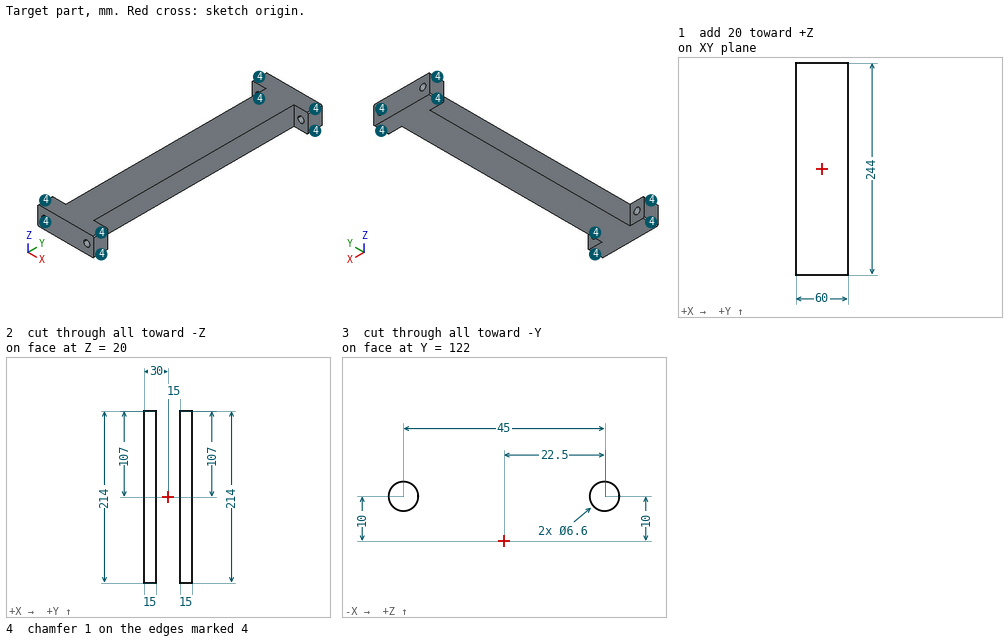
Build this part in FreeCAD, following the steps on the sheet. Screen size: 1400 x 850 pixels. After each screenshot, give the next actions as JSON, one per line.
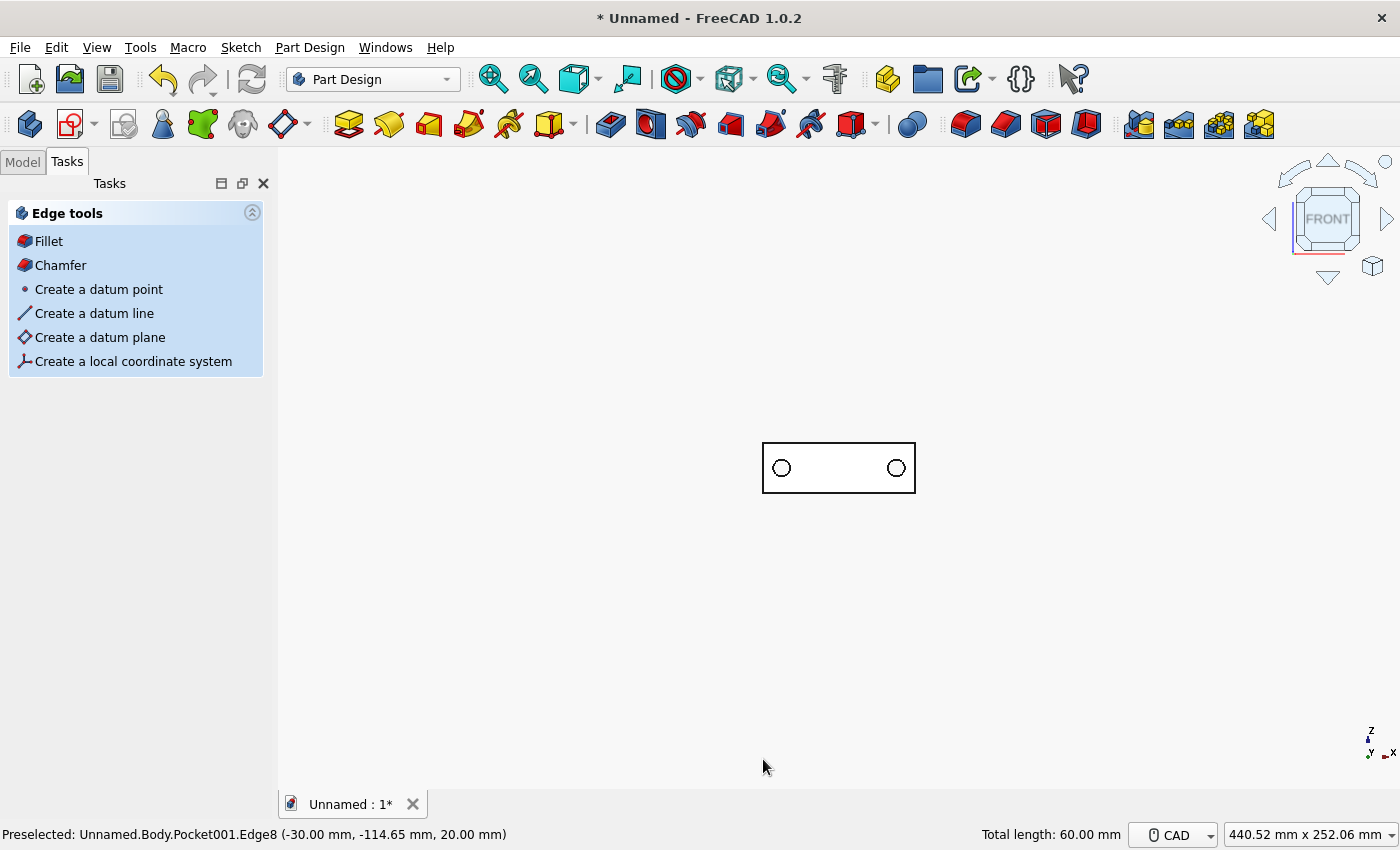
{"action": "left_click", "coordinate": [494, 80]}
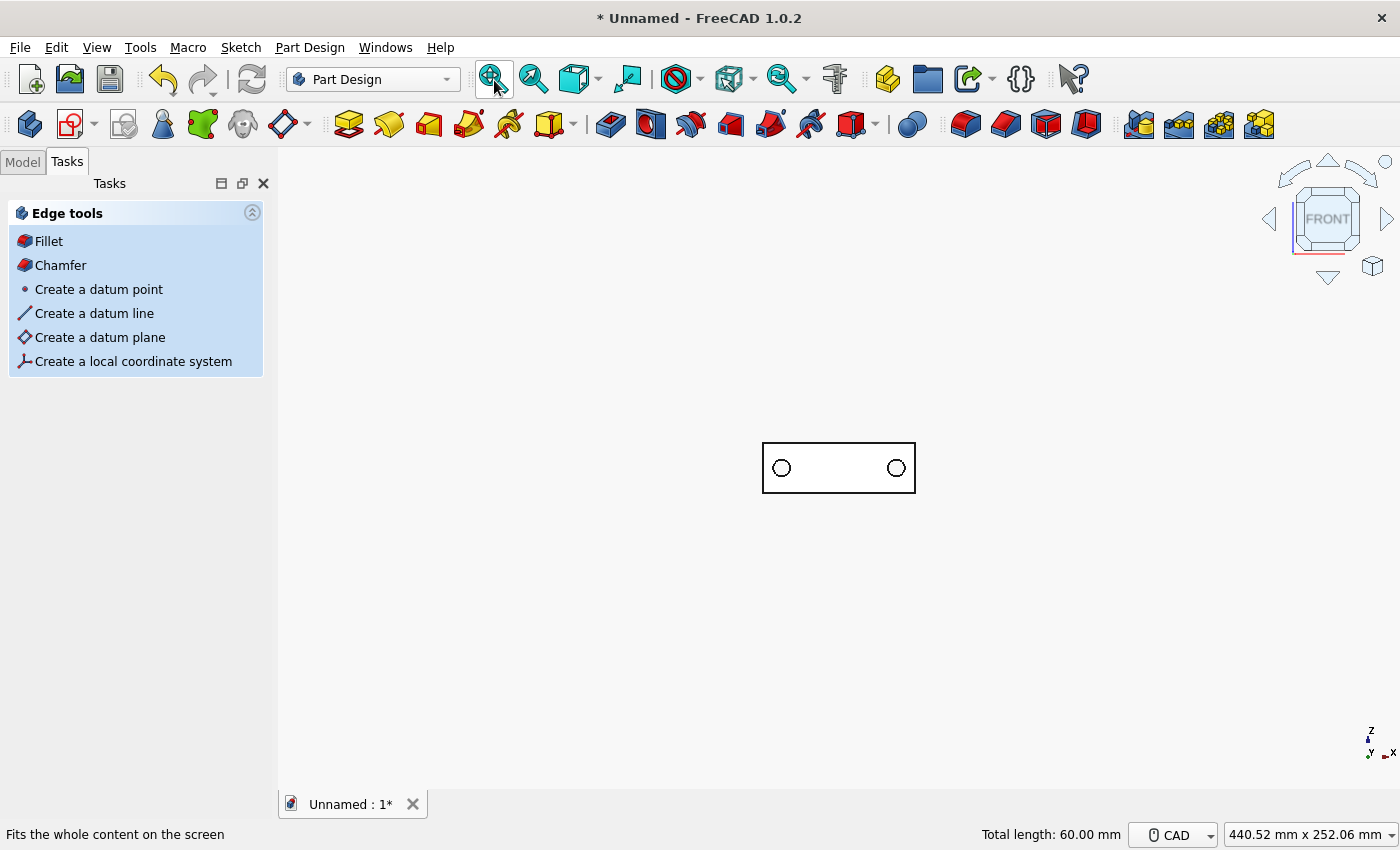
{"action": "key", "text": "3"}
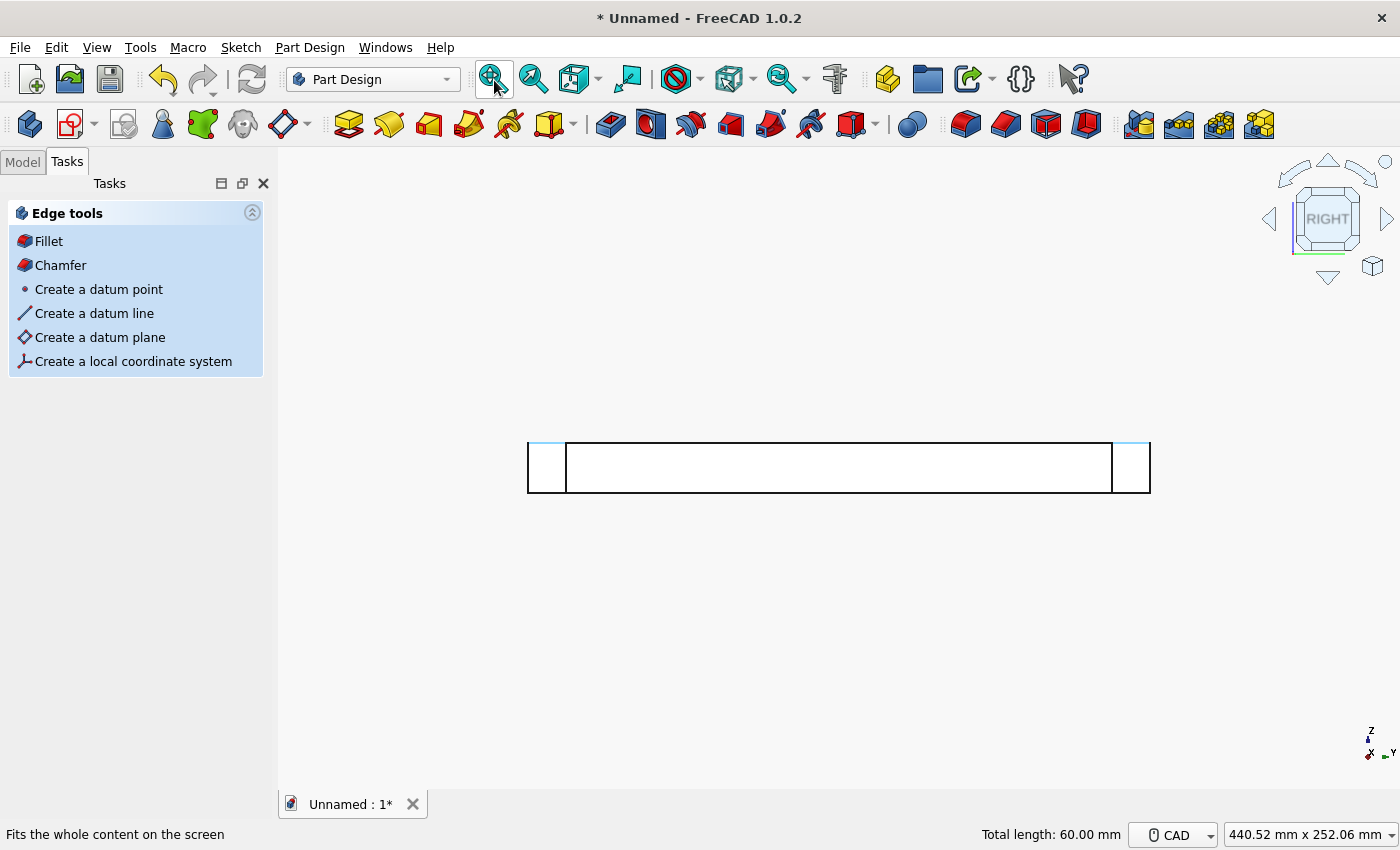
{"action": "left_click", "coordinate": [1131, 492], "text": "ctrl"}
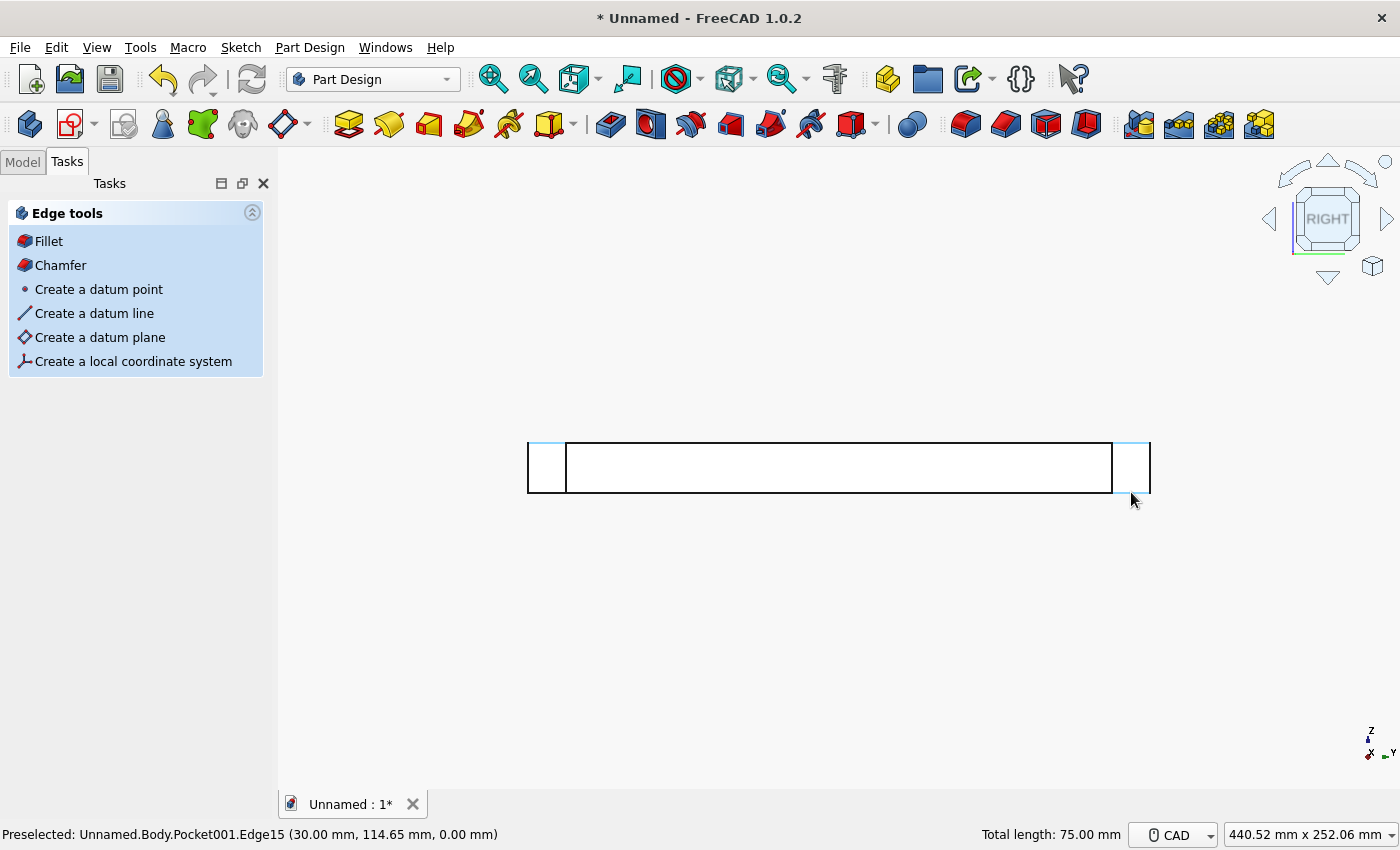
{"action": "left_click", "coordinate": [547, 492], "text": "ctrl"}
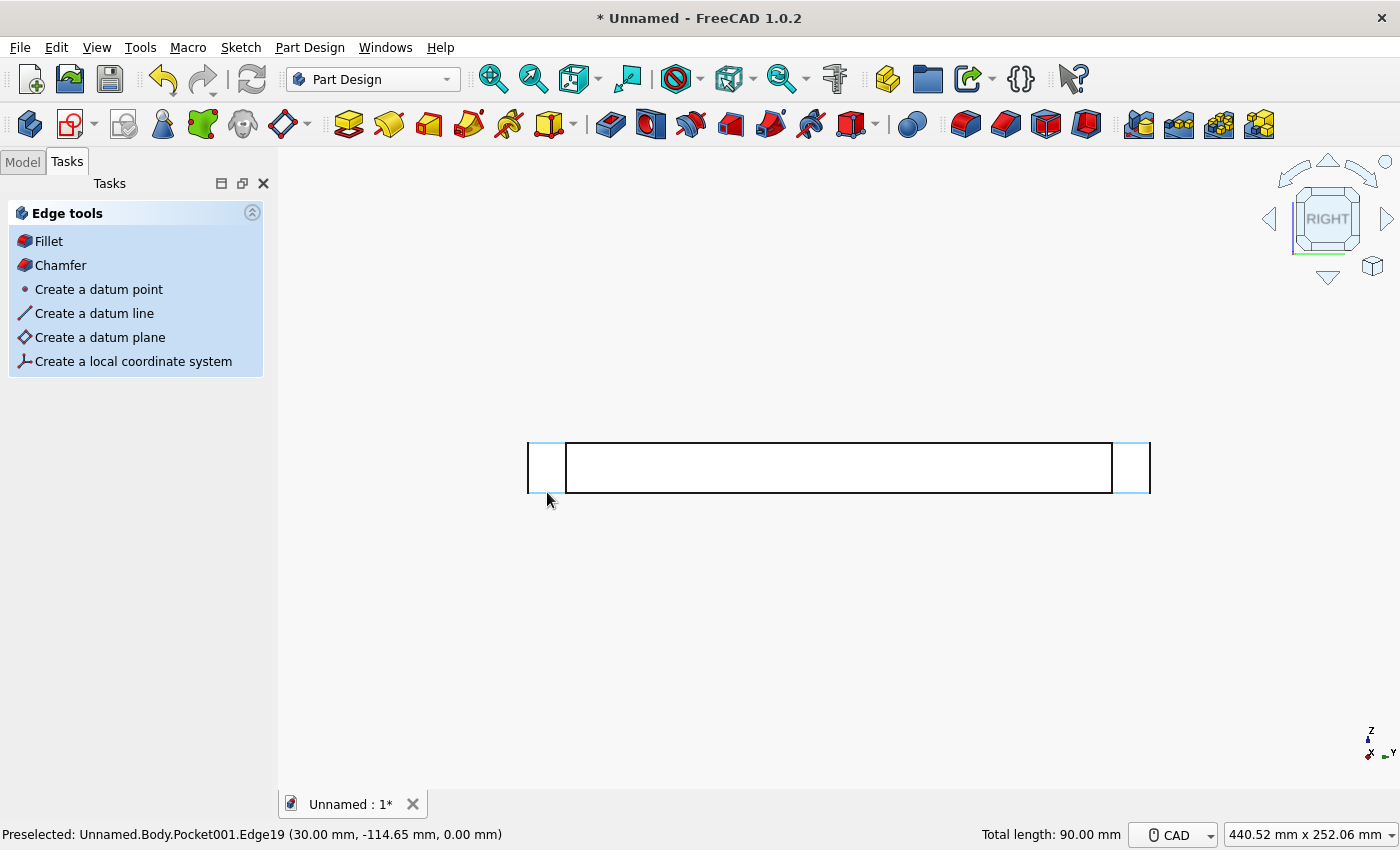
{"action": "key", "text": "5"}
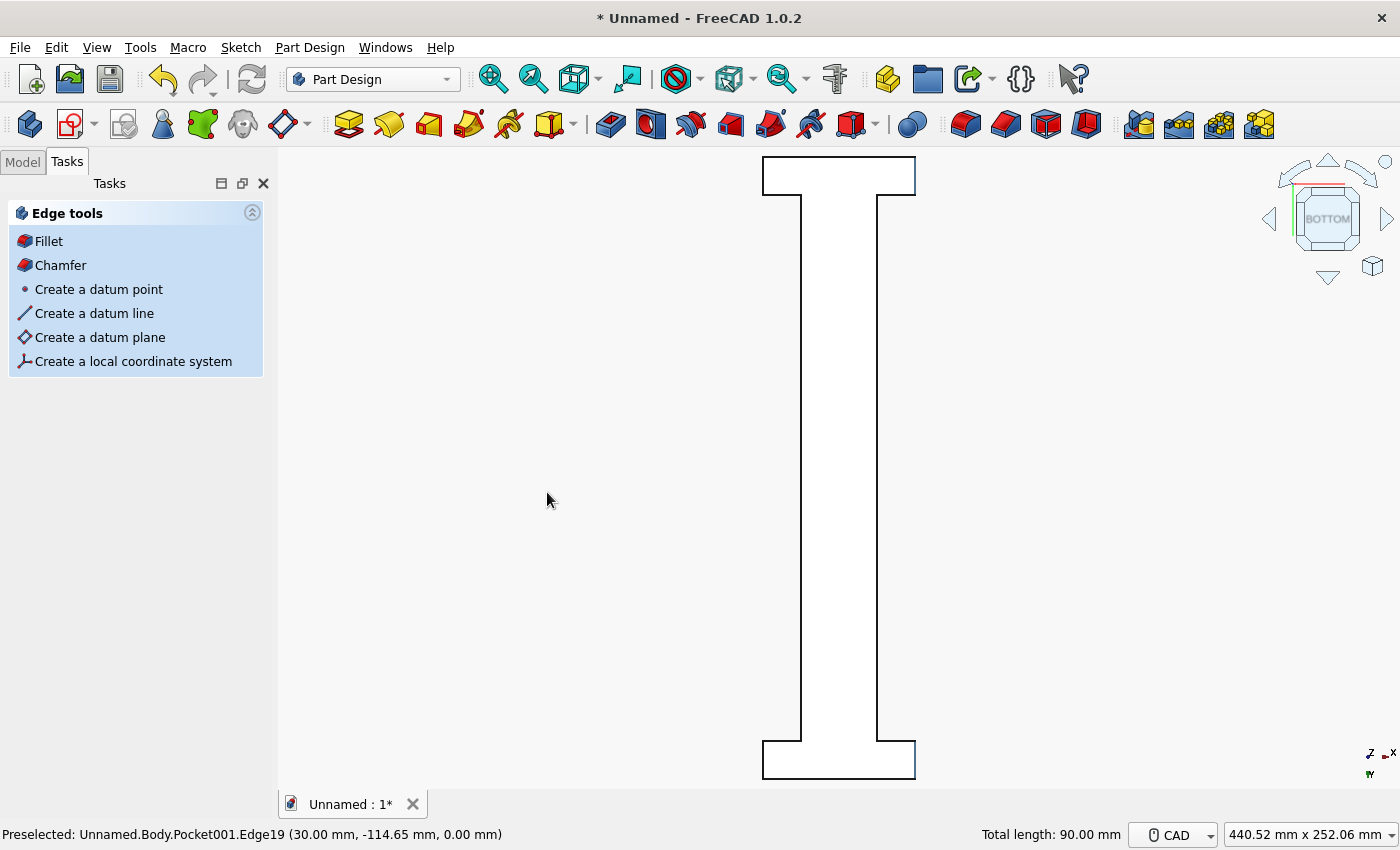
{"action": "left_click", "coordinate": [763, 179], "text": "ctrl"}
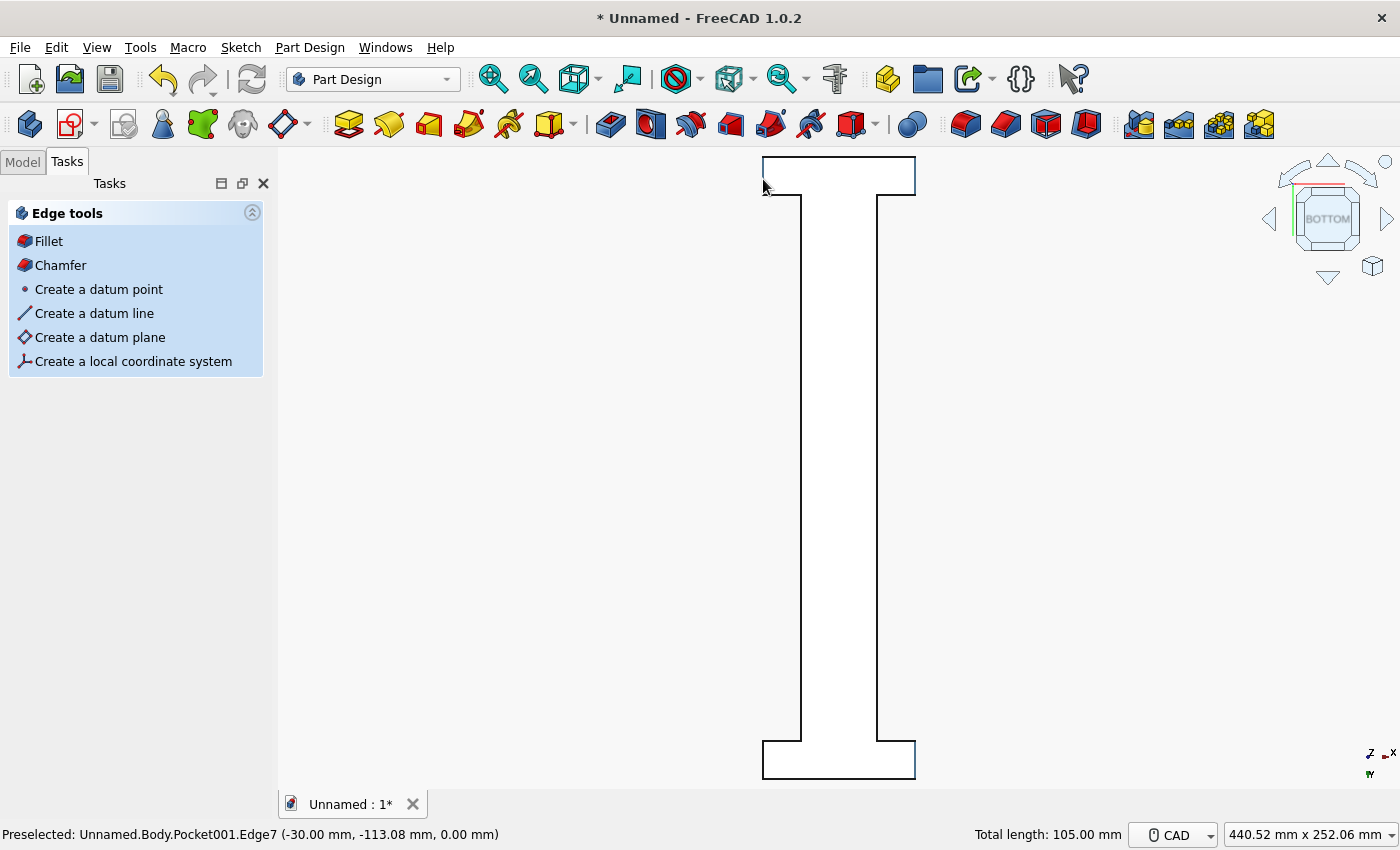
{"action": "left_click", "coordinate": [763, 759], "text": "ctrl"}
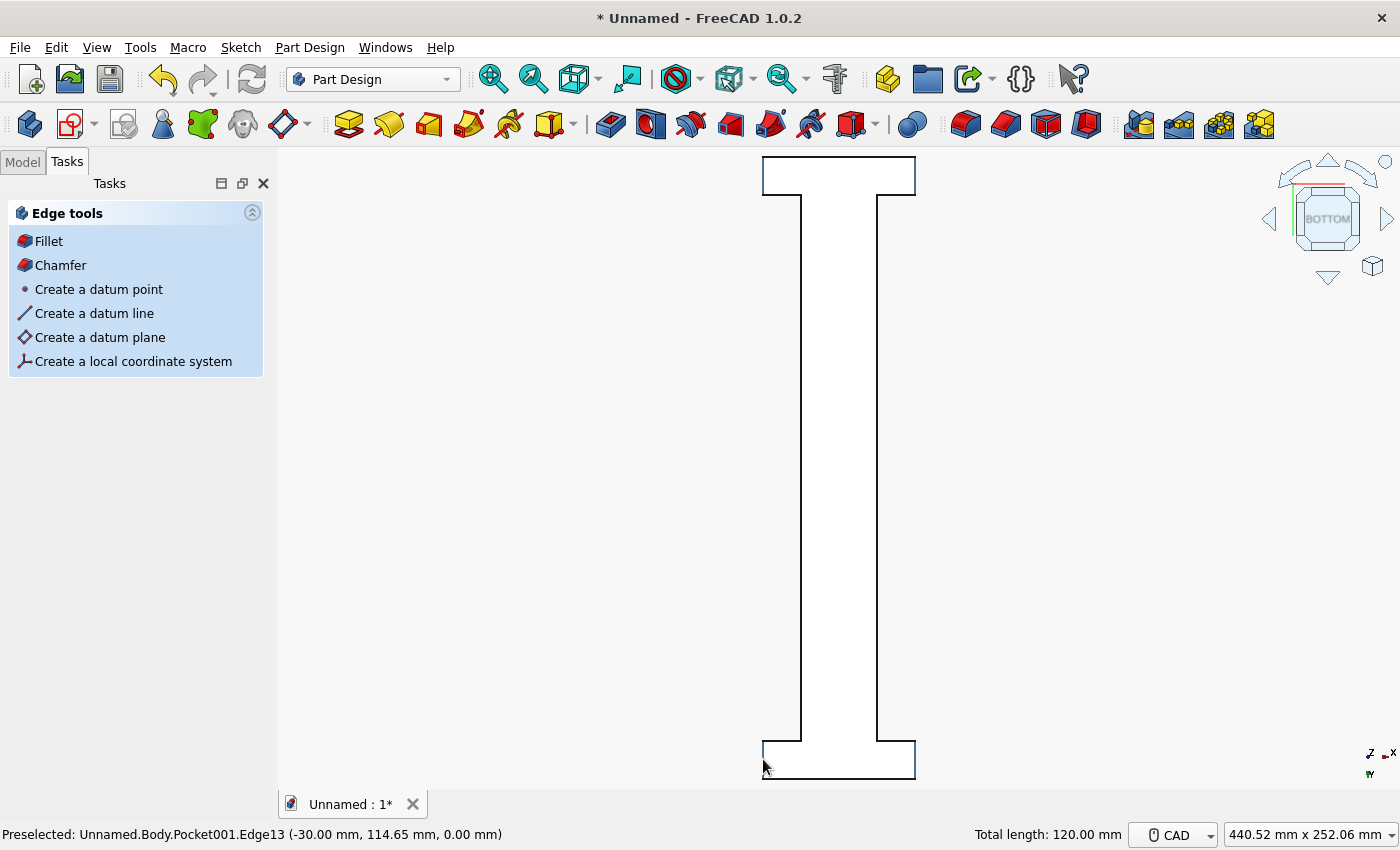
{"action": "left_click", "coordinate": [1006, 124]}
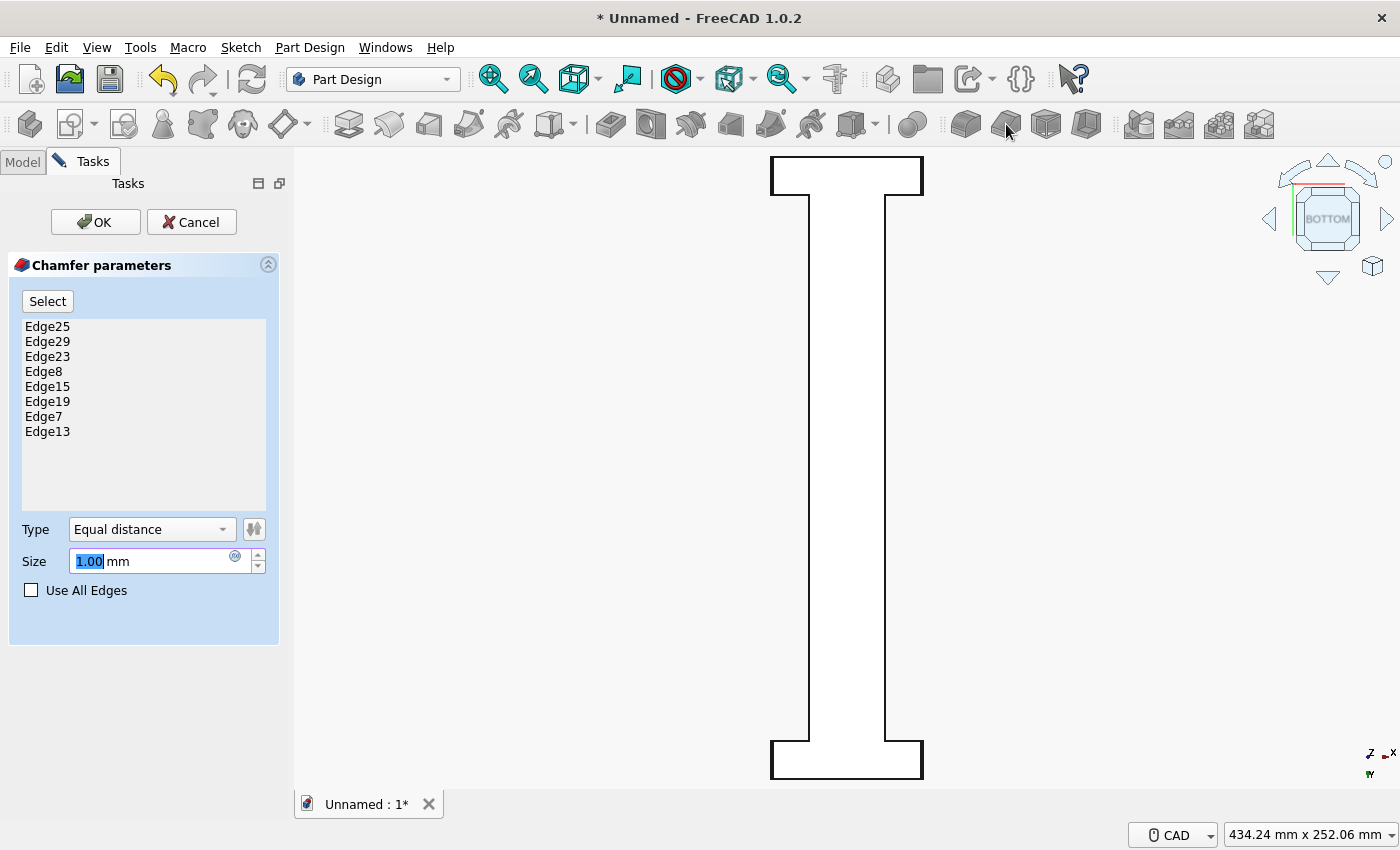
{"action": "type", "text": "1"}
{"action": "key", "text": "Tab"}